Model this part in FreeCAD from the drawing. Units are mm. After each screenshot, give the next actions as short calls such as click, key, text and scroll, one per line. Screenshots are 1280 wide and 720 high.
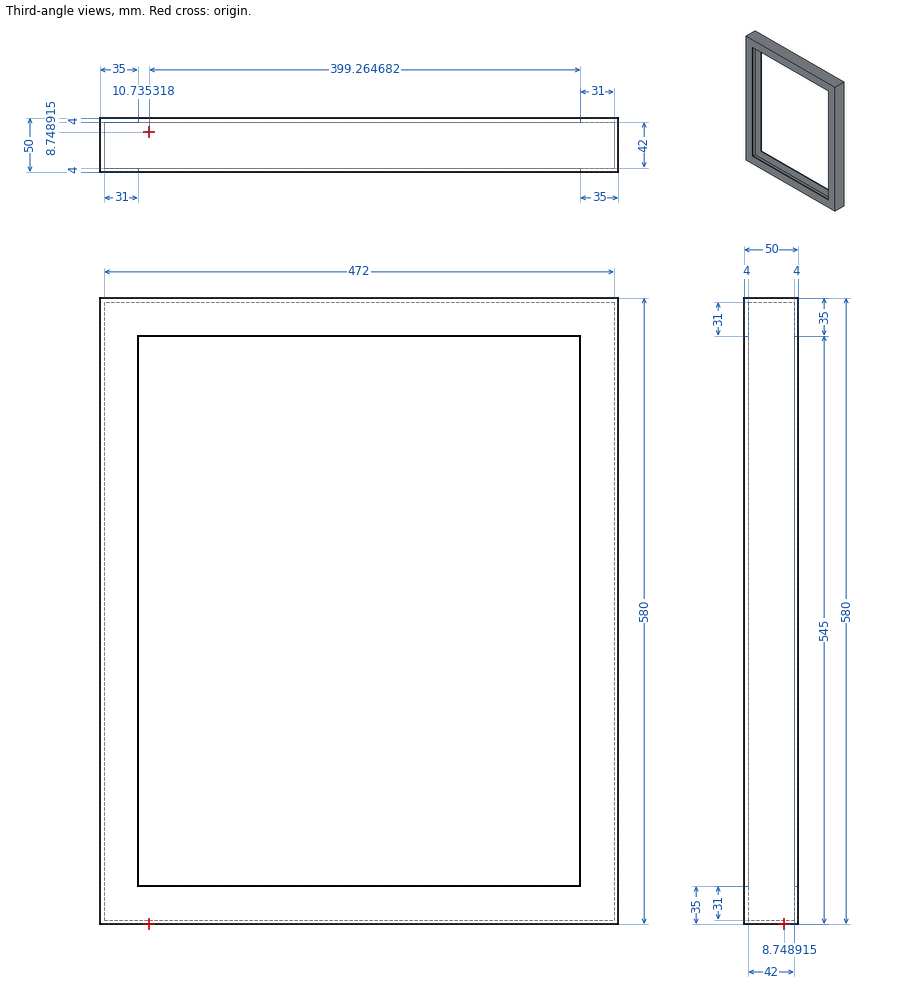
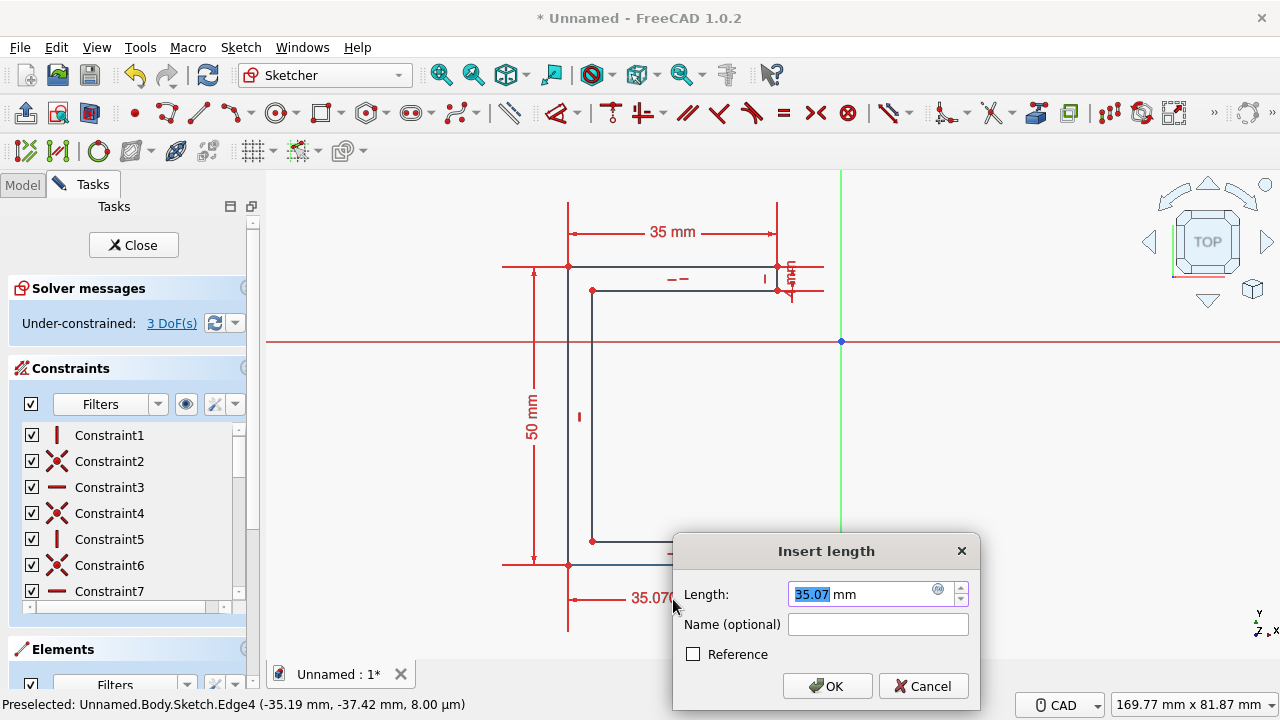
text(35)
key(Return)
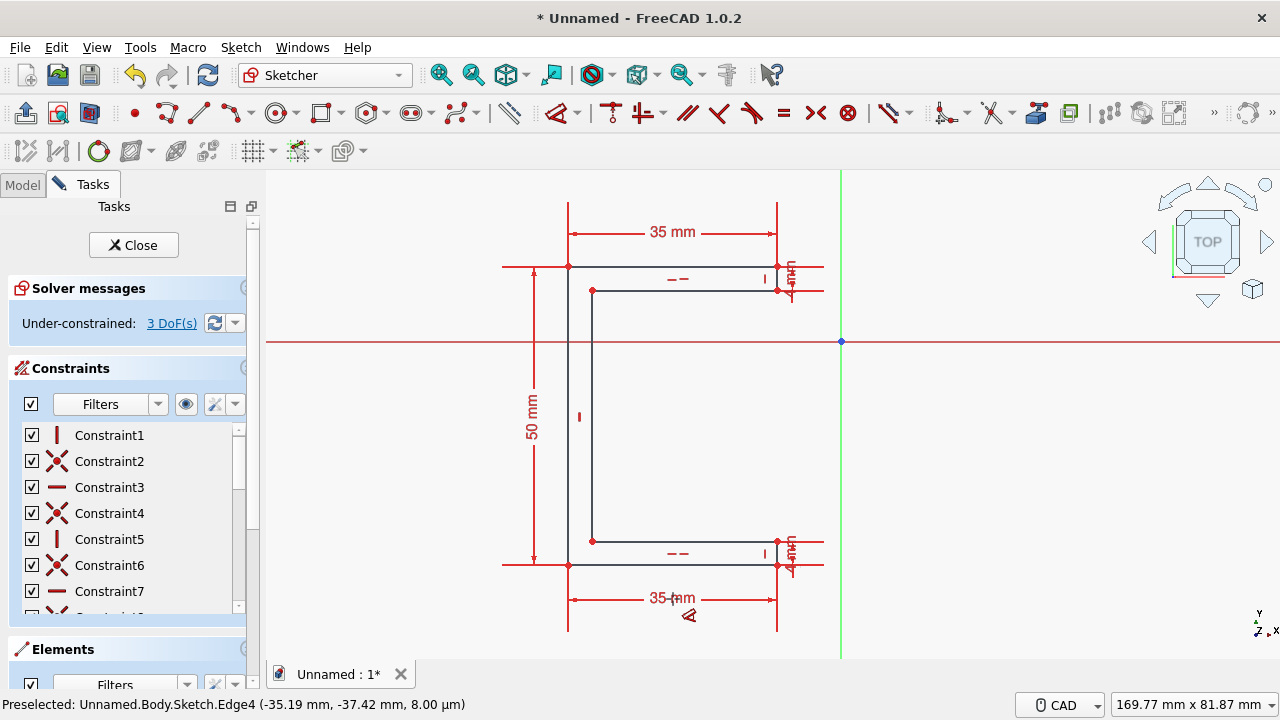
click(722, 542)
click(685, 508)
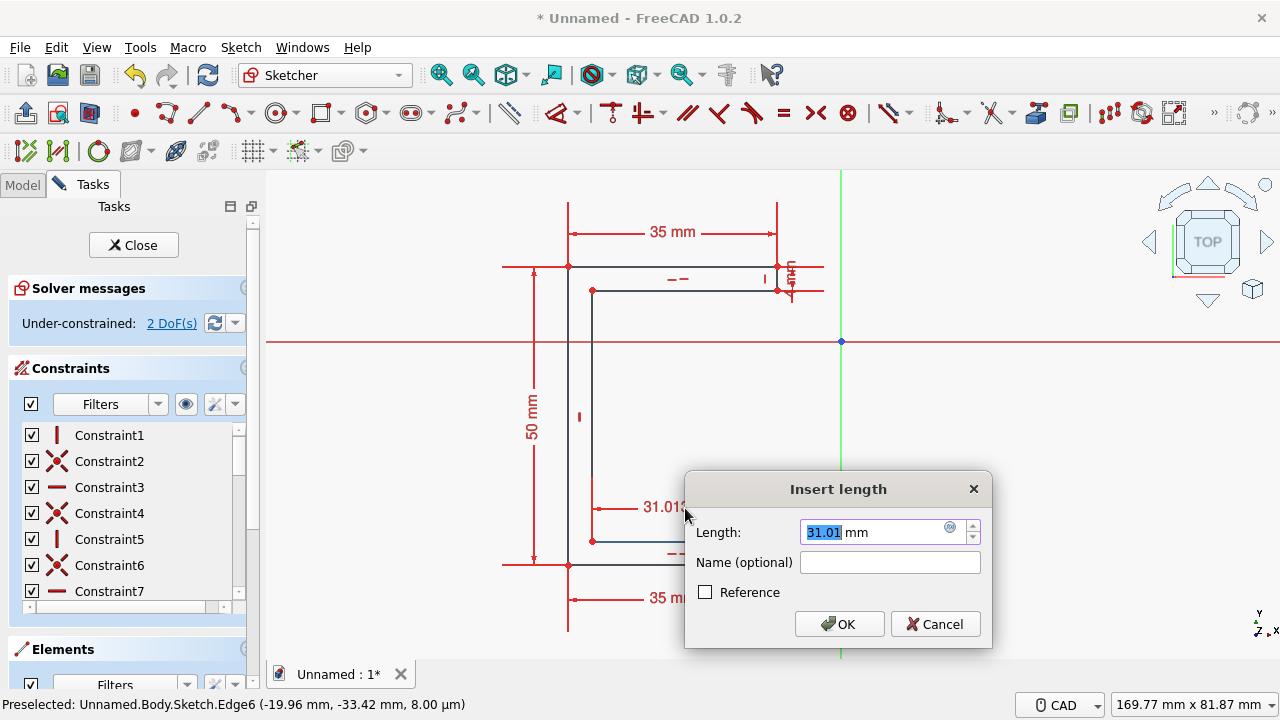
text(31)
key(Return)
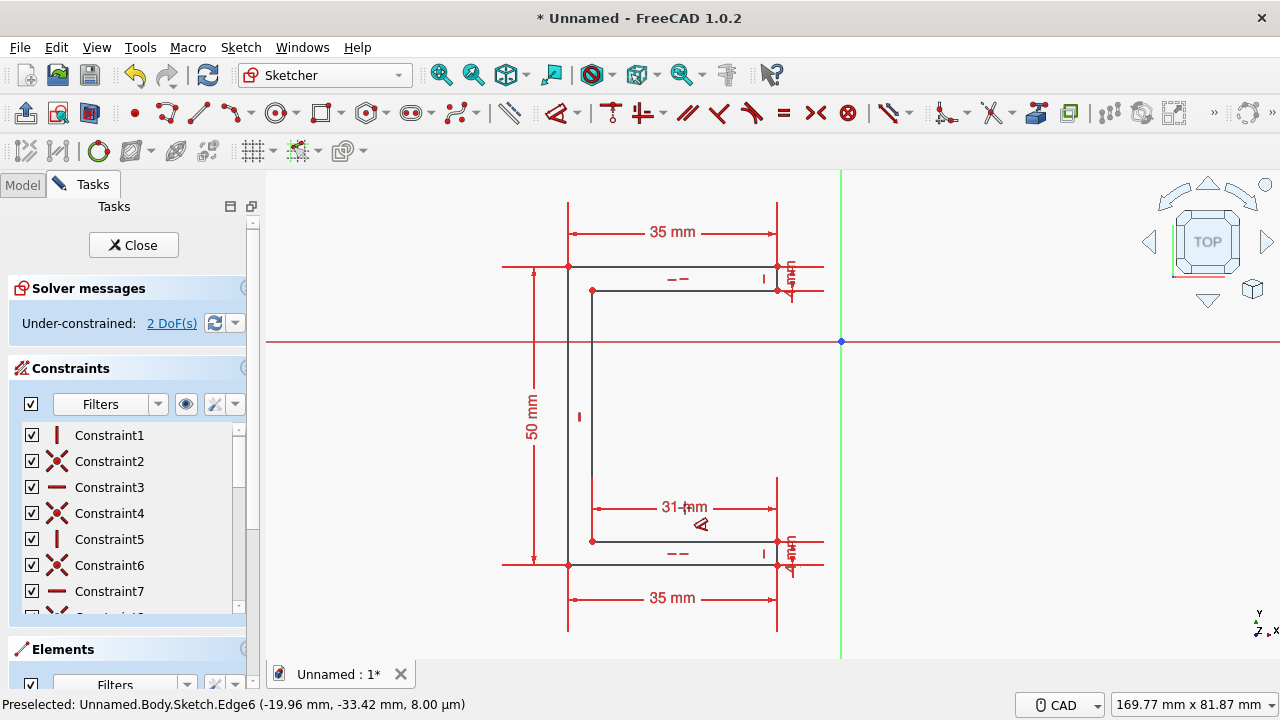
click(777, 291)
click(875, 316)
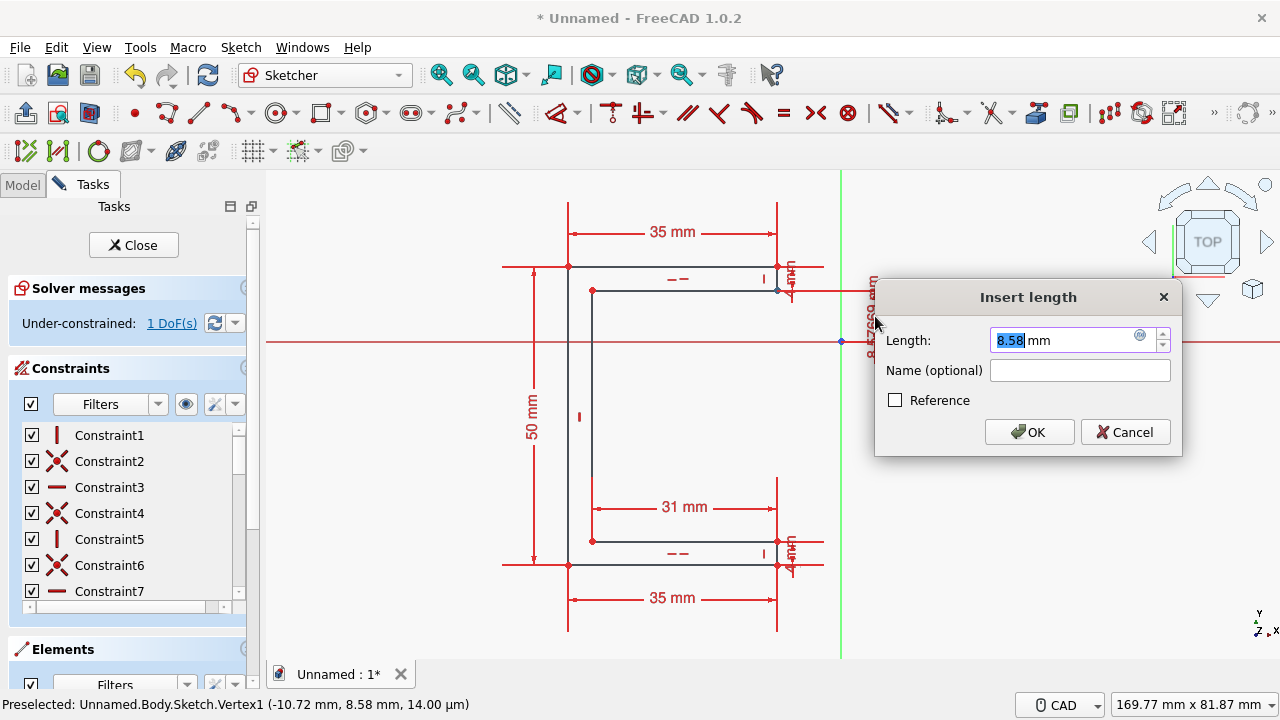
text(8.748915)
key(Return)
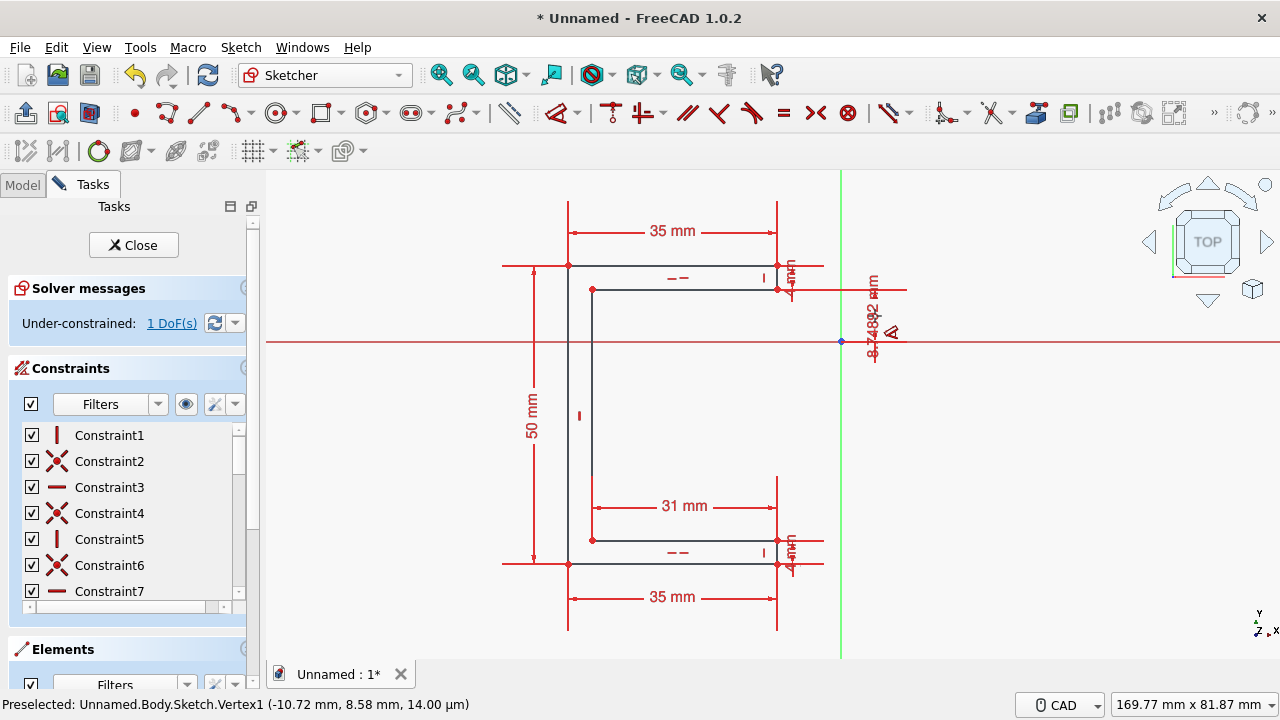
click(777, 290)
click(809, 256)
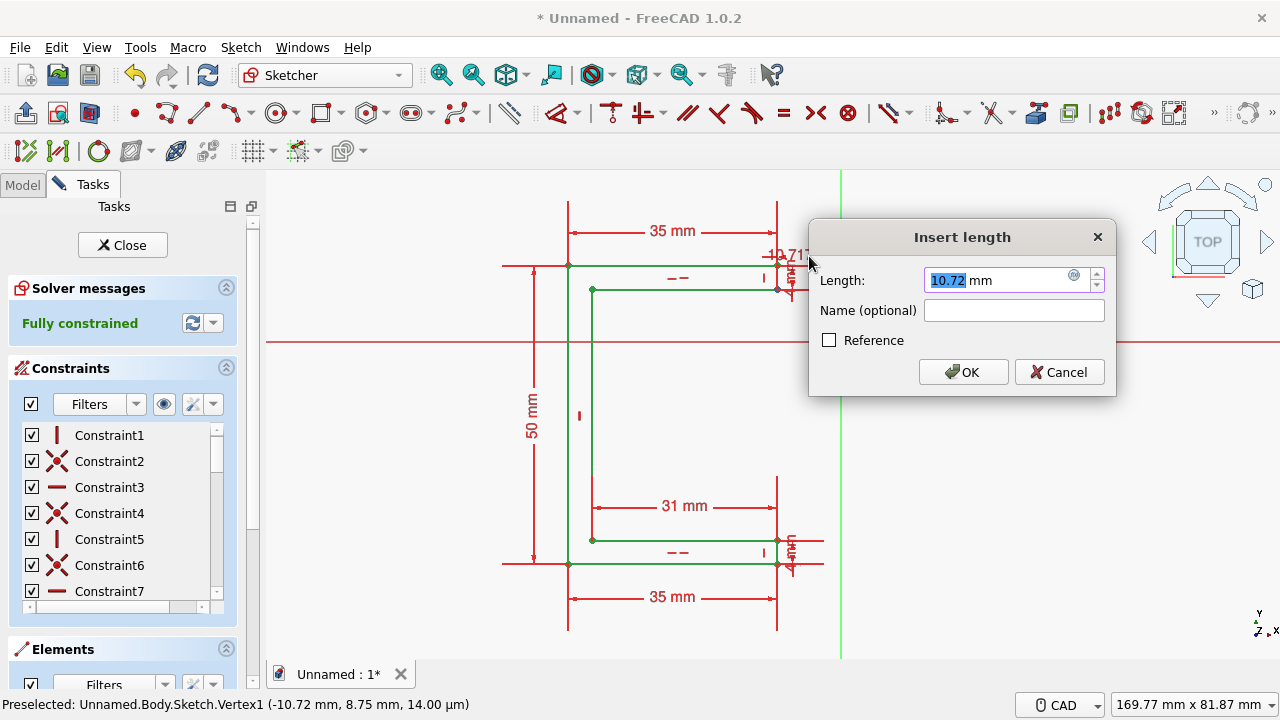
text(10.735318)
key(Return)
key(Escape)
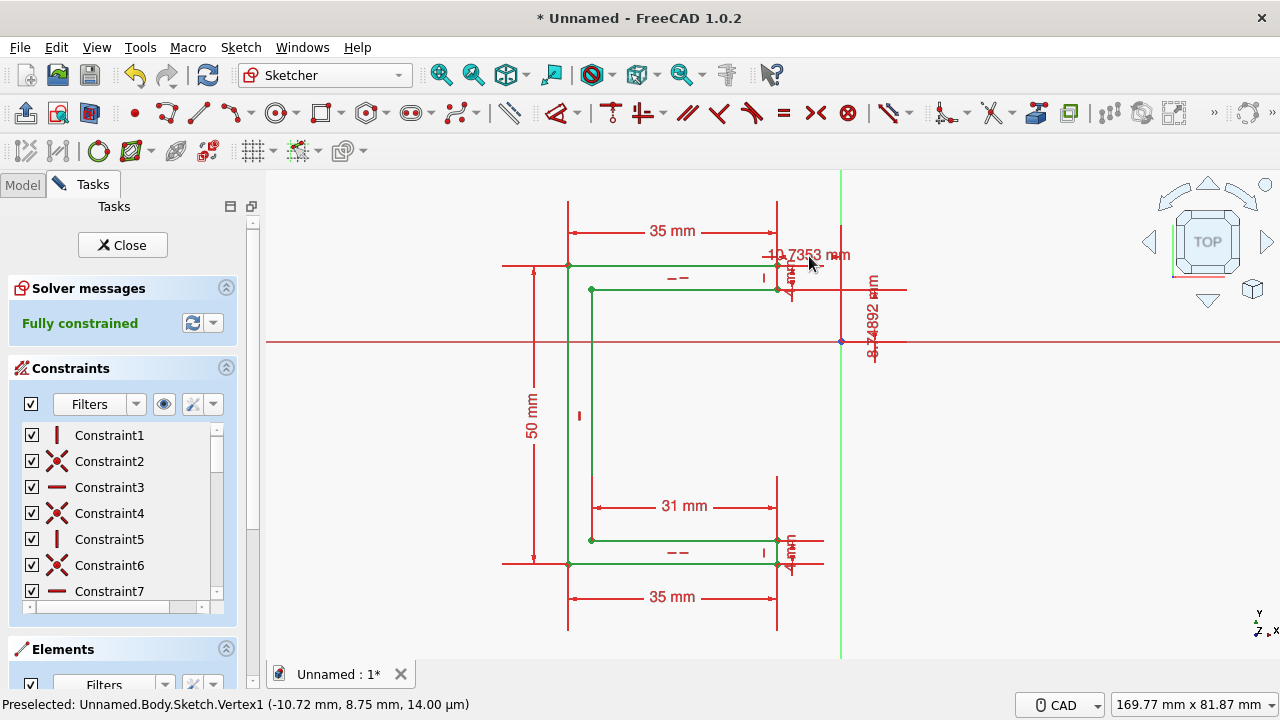
click(123, 245)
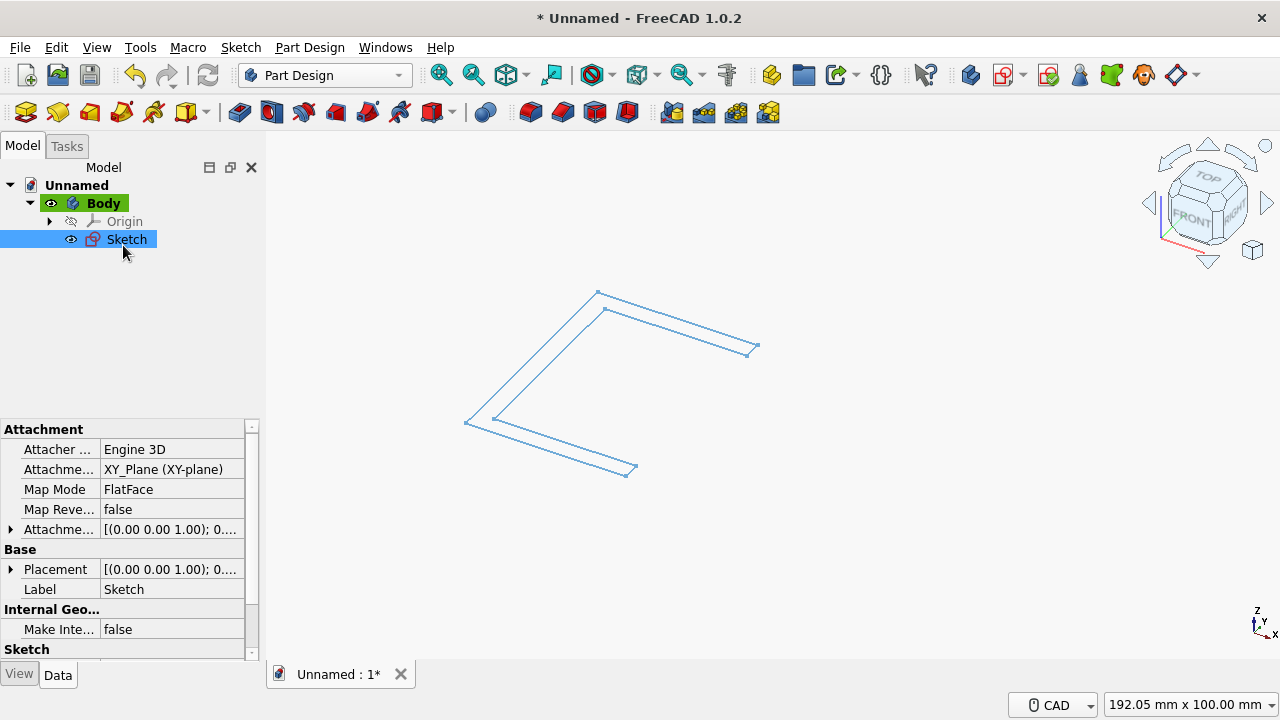
click(26, 112)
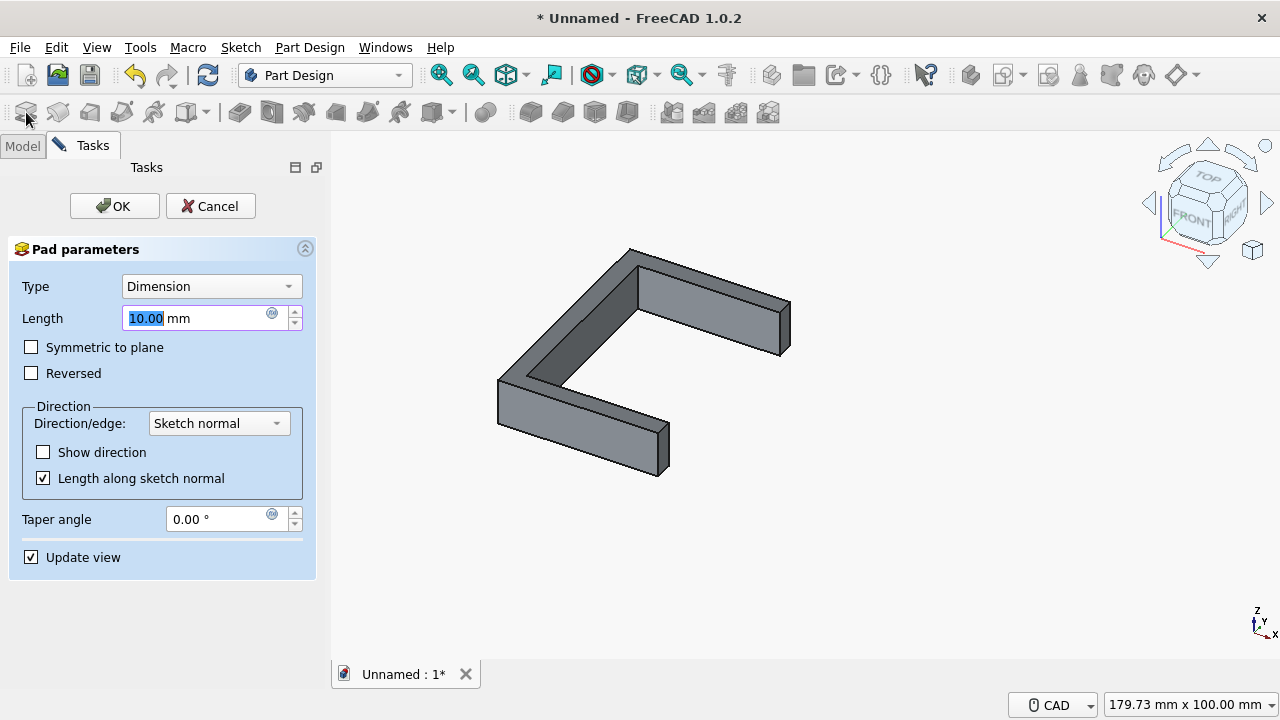
text(580)
key(Tab)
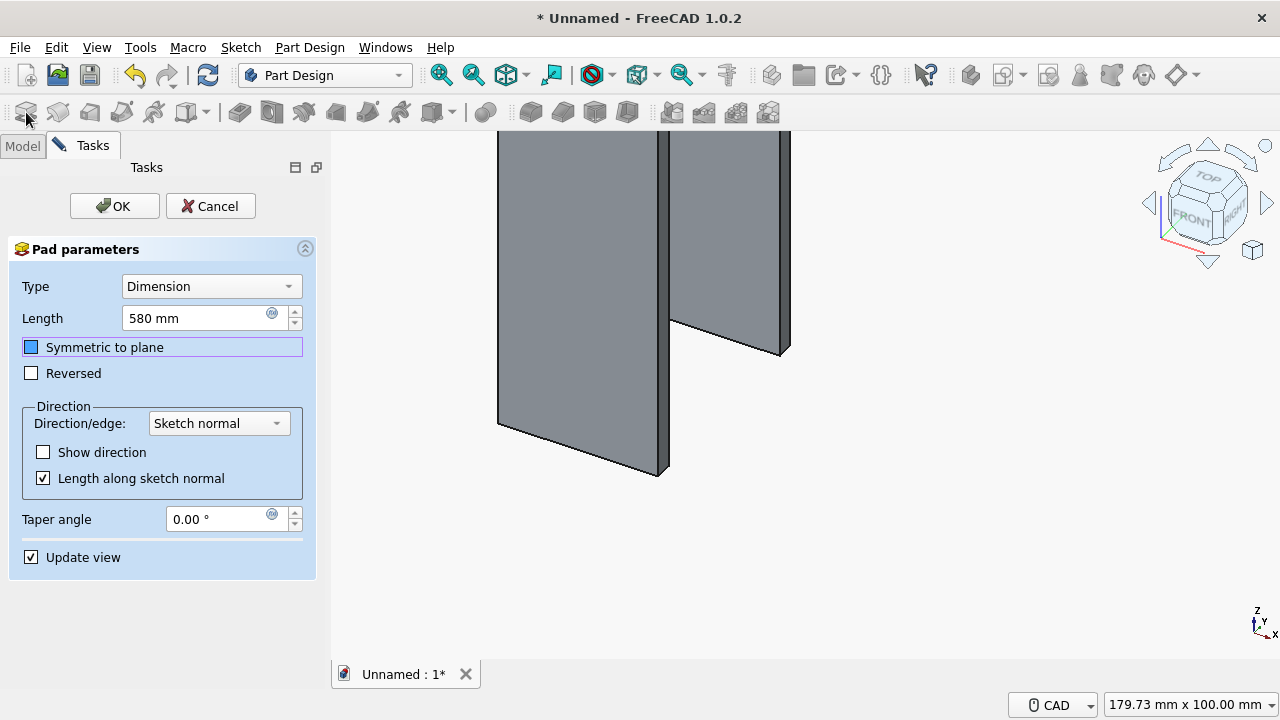
click(115, 206)